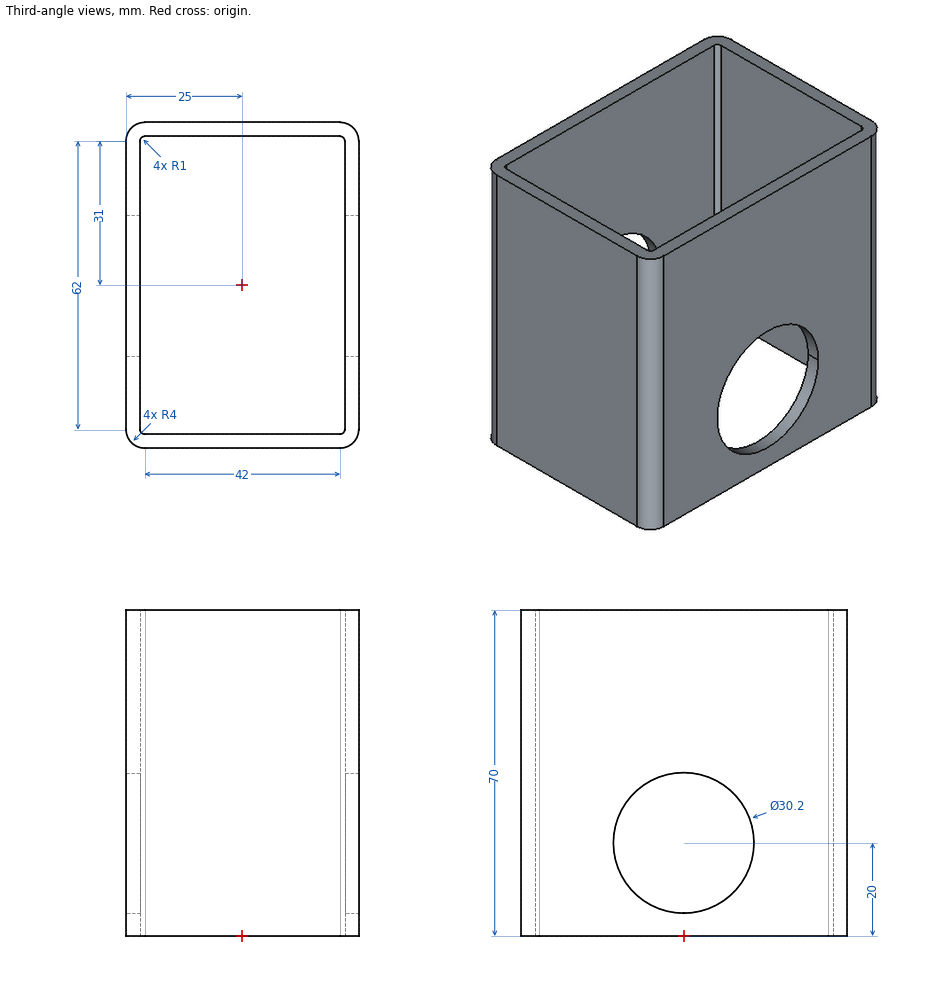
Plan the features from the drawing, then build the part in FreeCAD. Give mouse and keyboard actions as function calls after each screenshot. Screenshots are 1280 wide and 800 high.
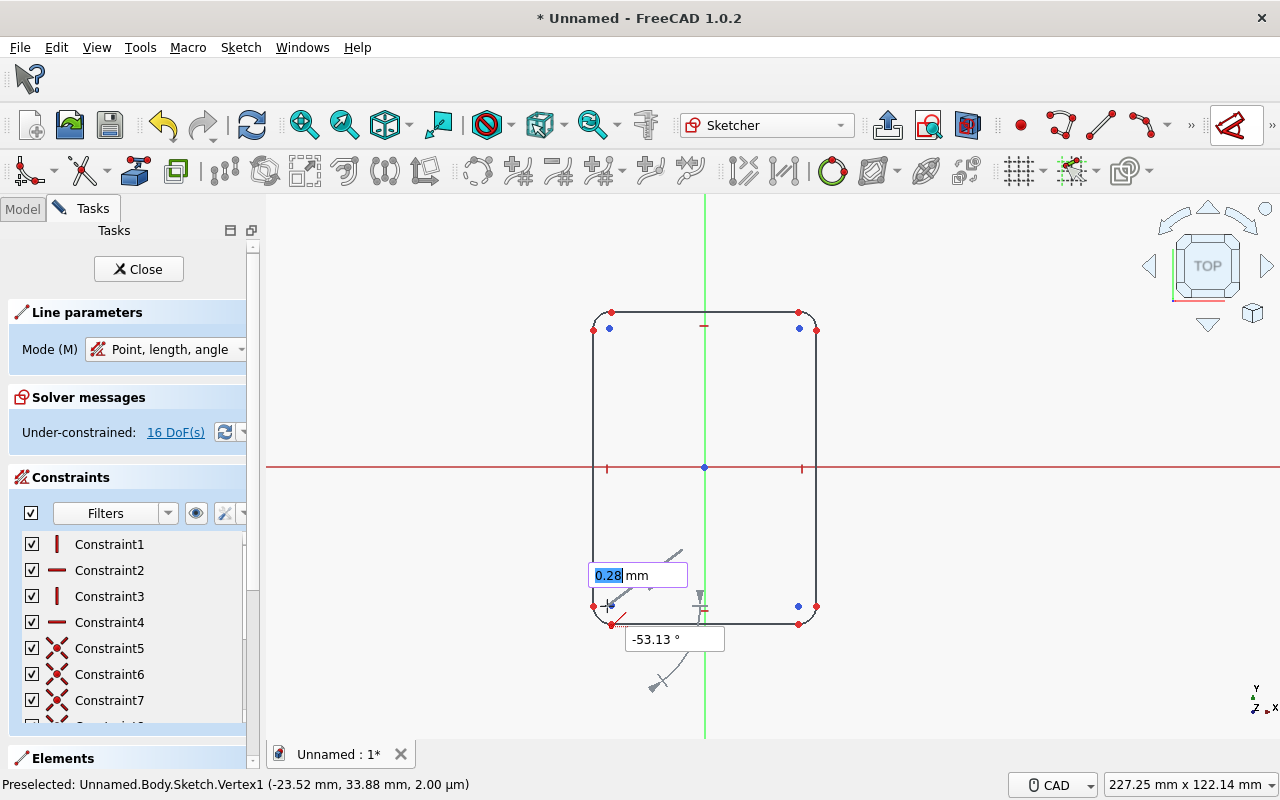
scroll(607, 329, up, 7)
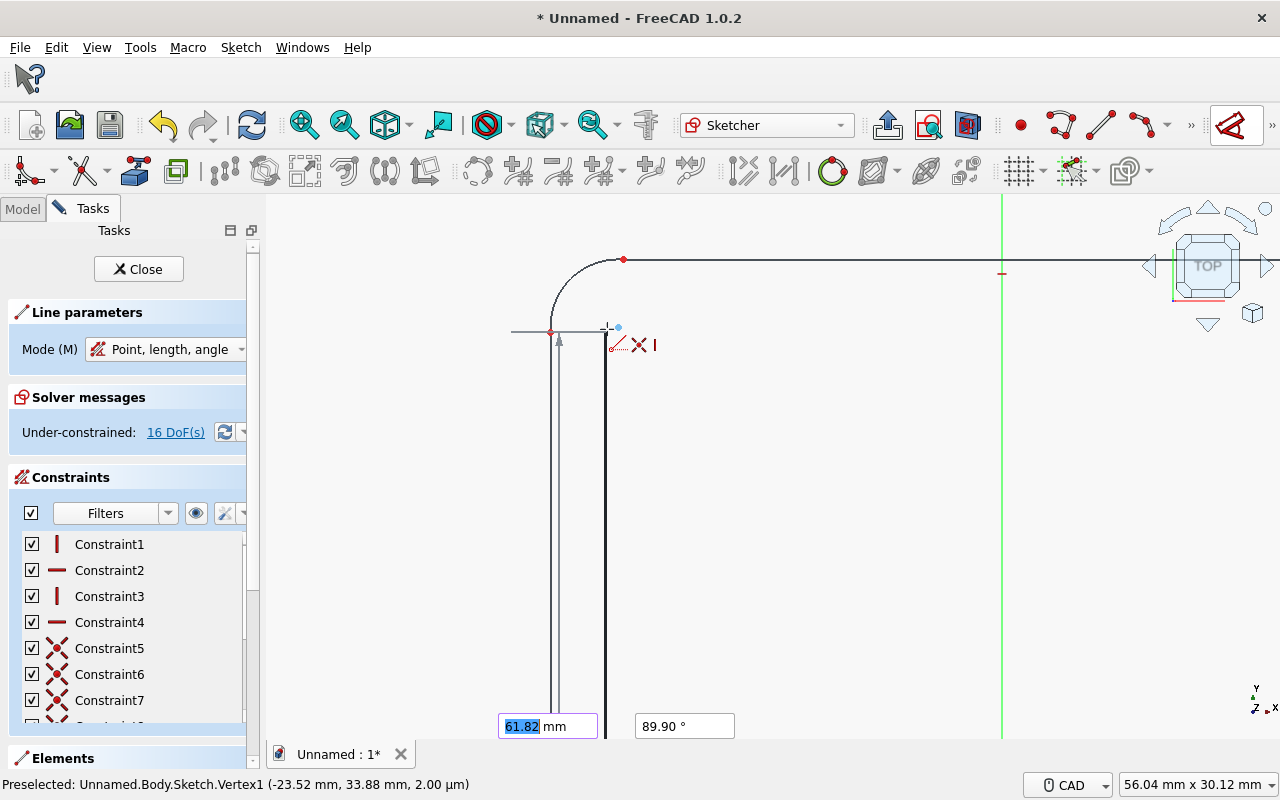
click(604, 328)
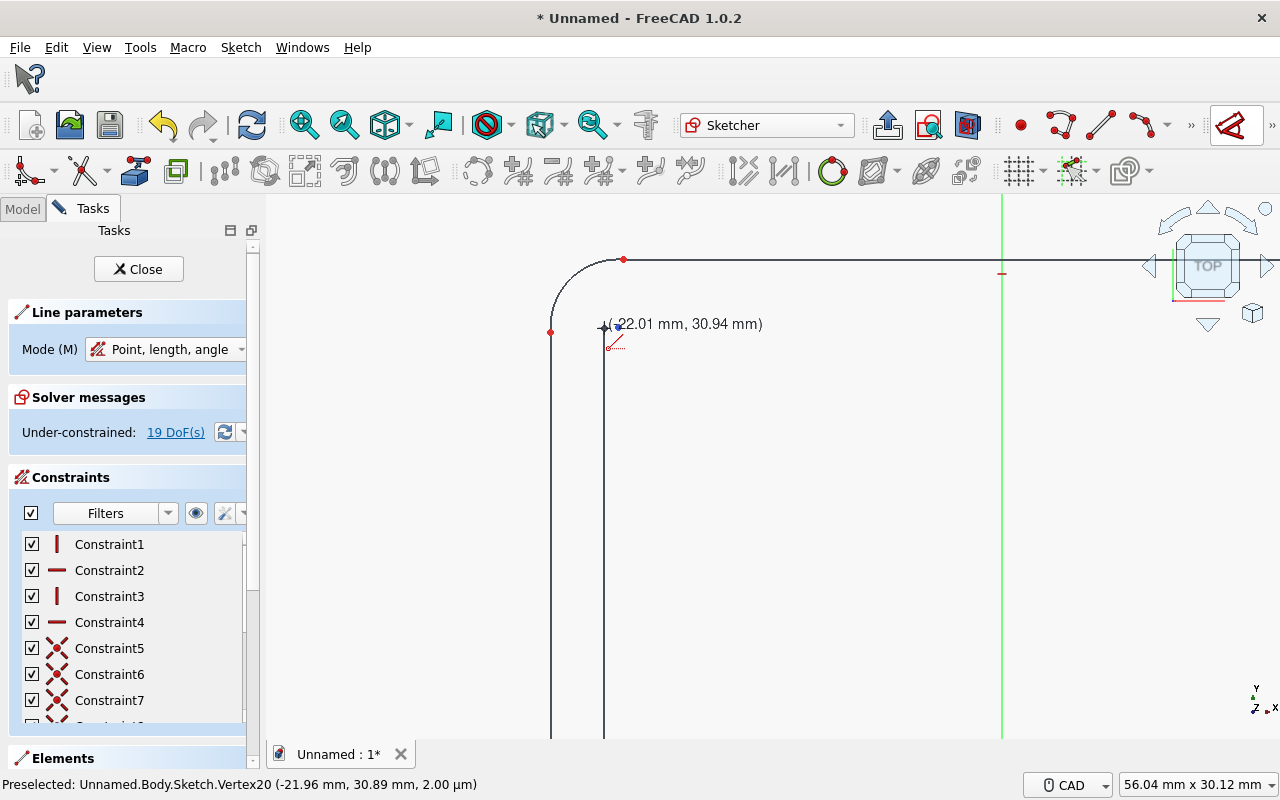
click(622, 310)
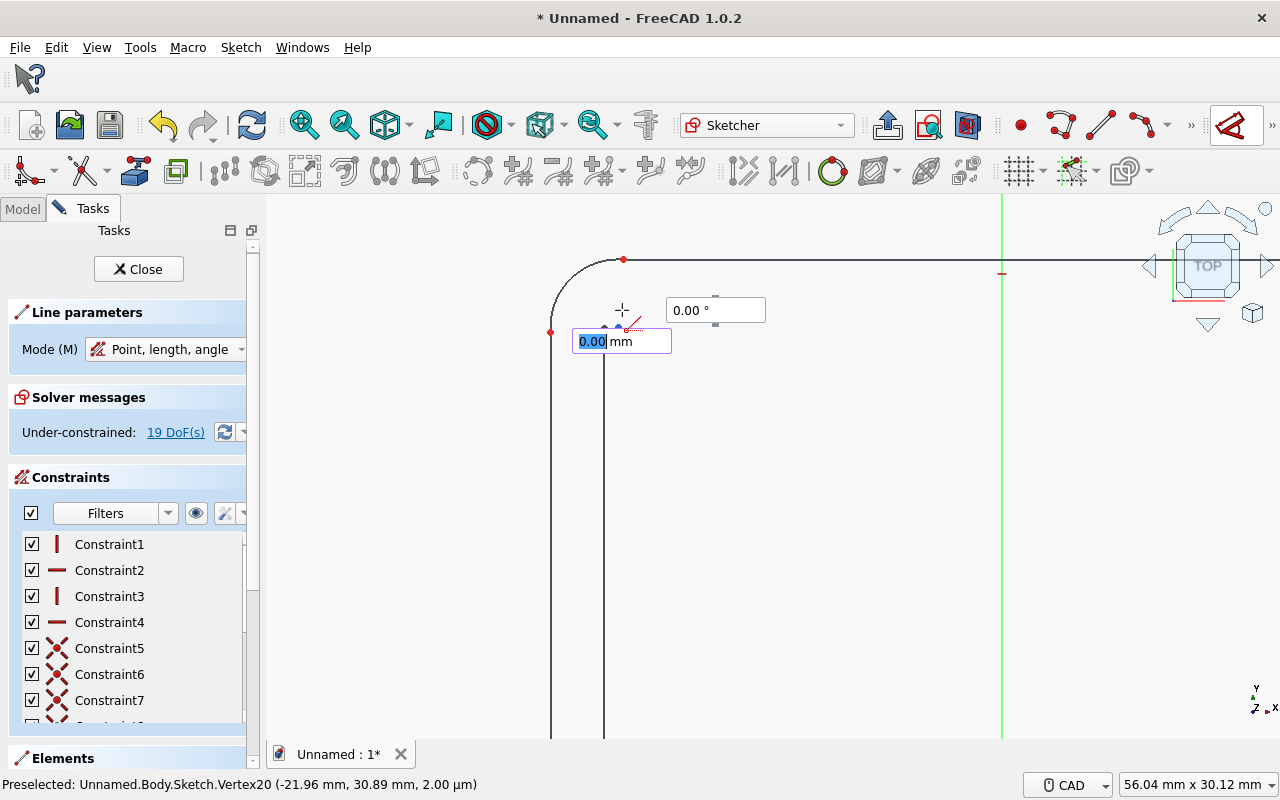
scroll(607, 328, down, 7)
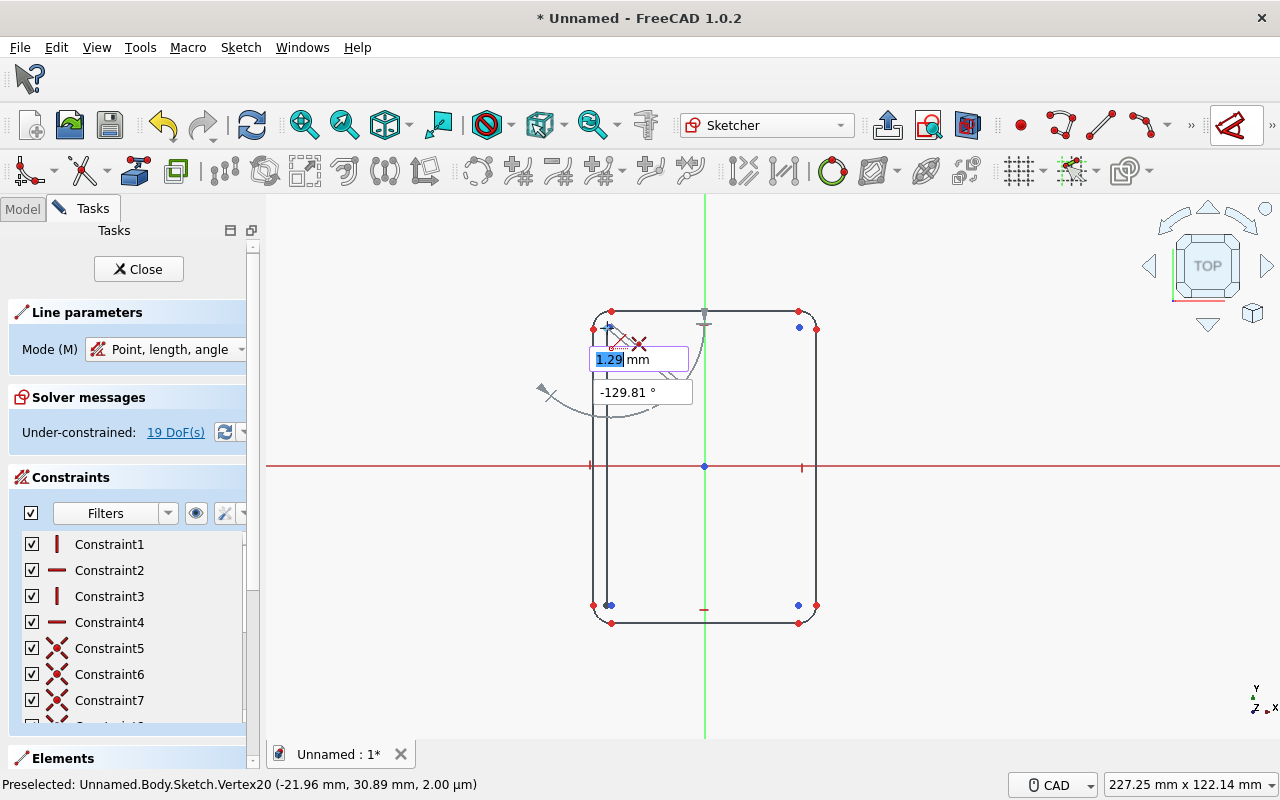
scroll(798, 324, up, 7)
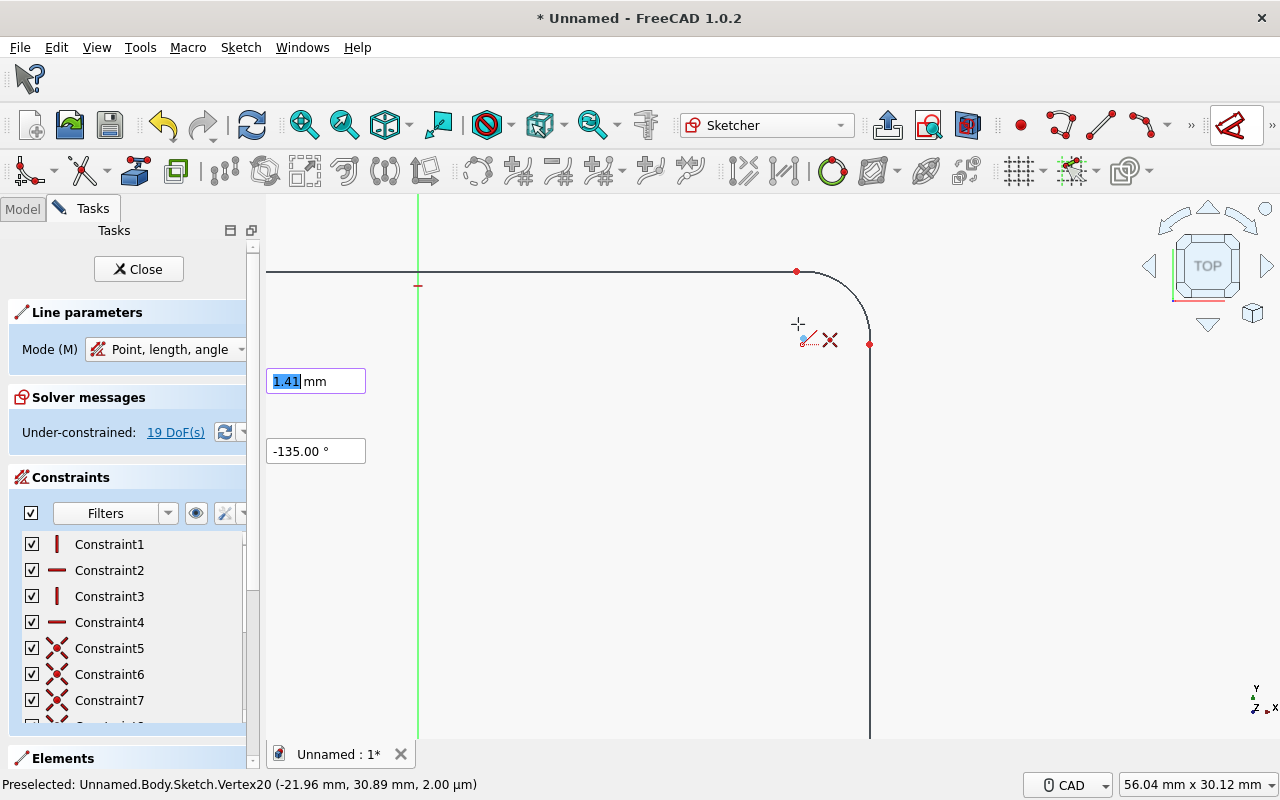
click(798, 322)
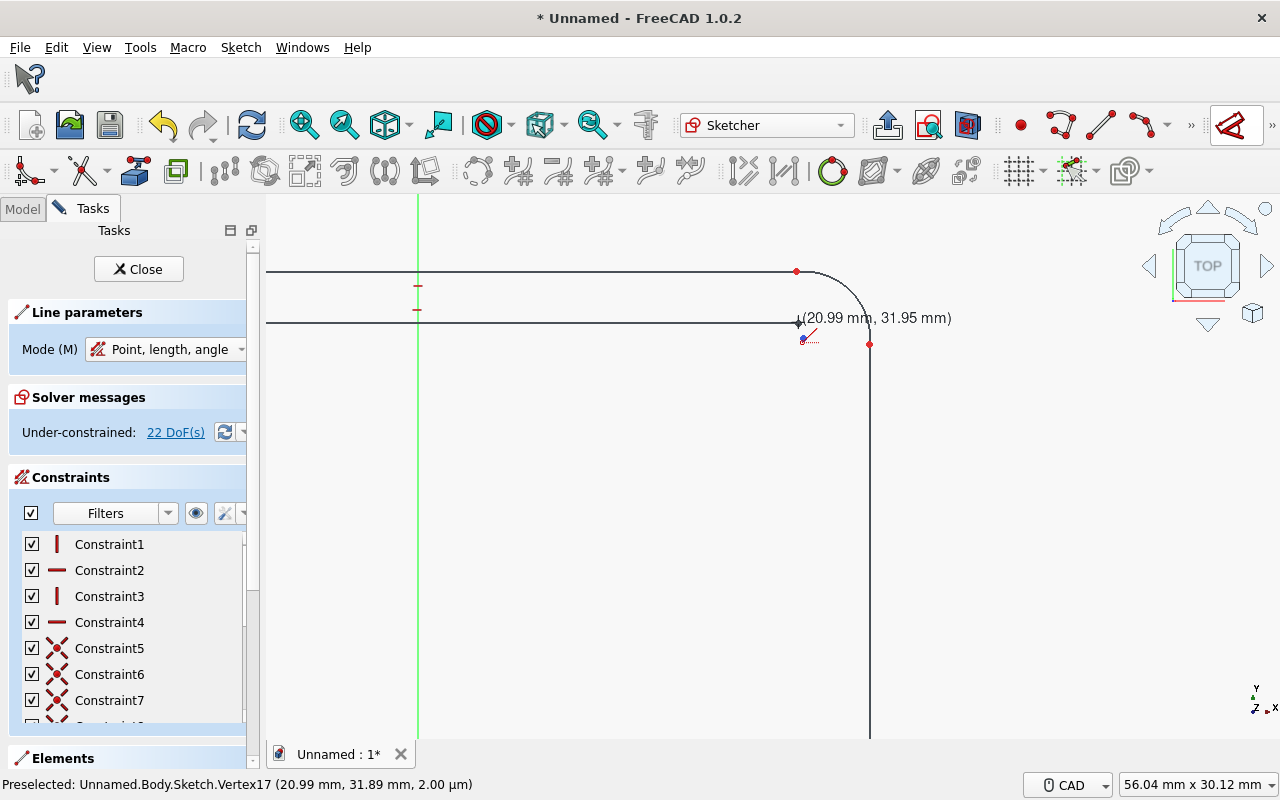
click(816, 340)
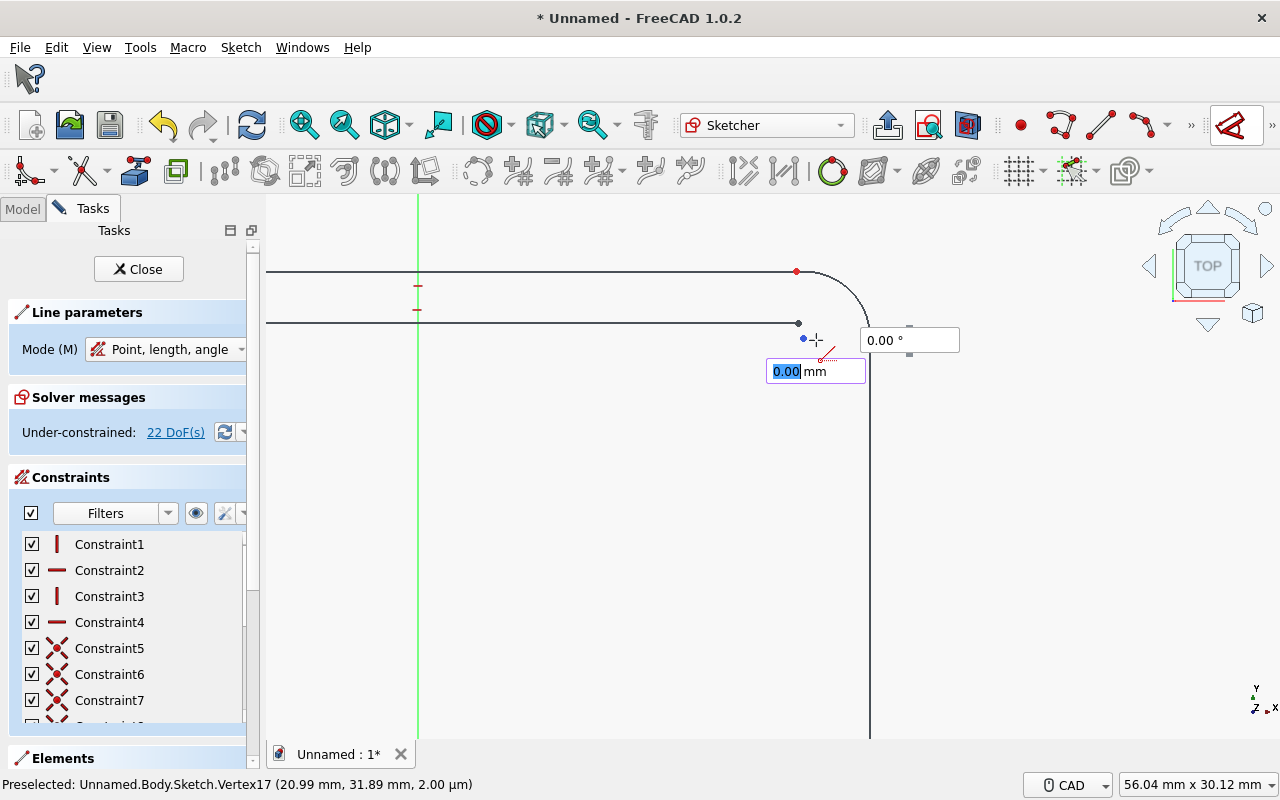
scroll(798, 324, down, 7)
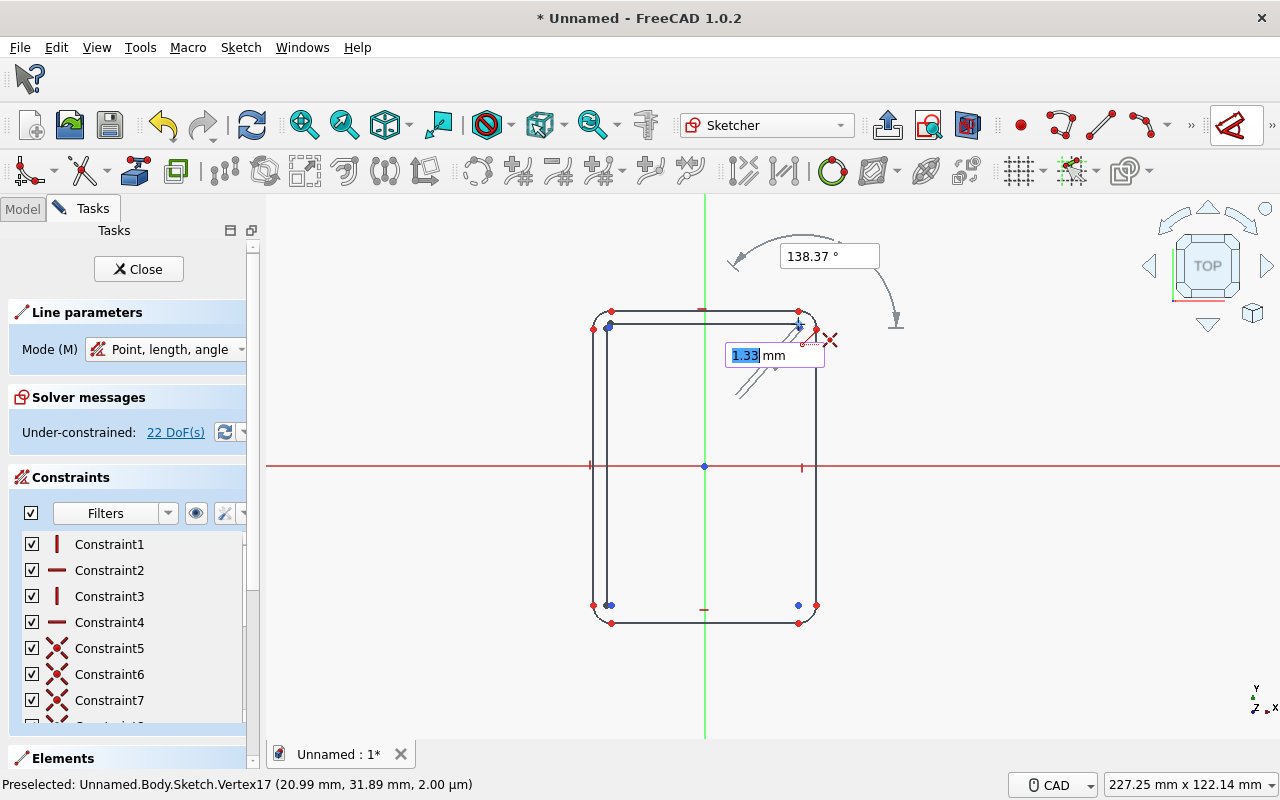
scroll(803, 605, up, 7)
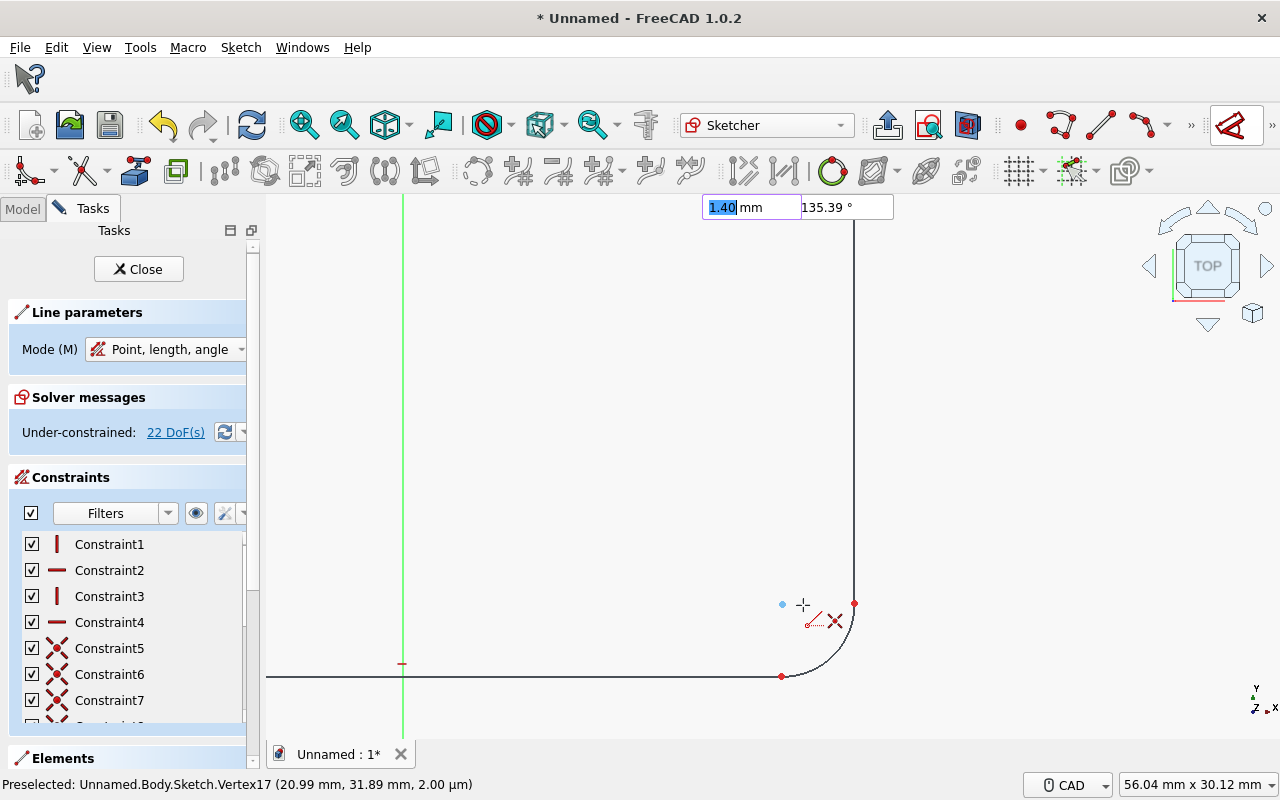
click(801, 602)